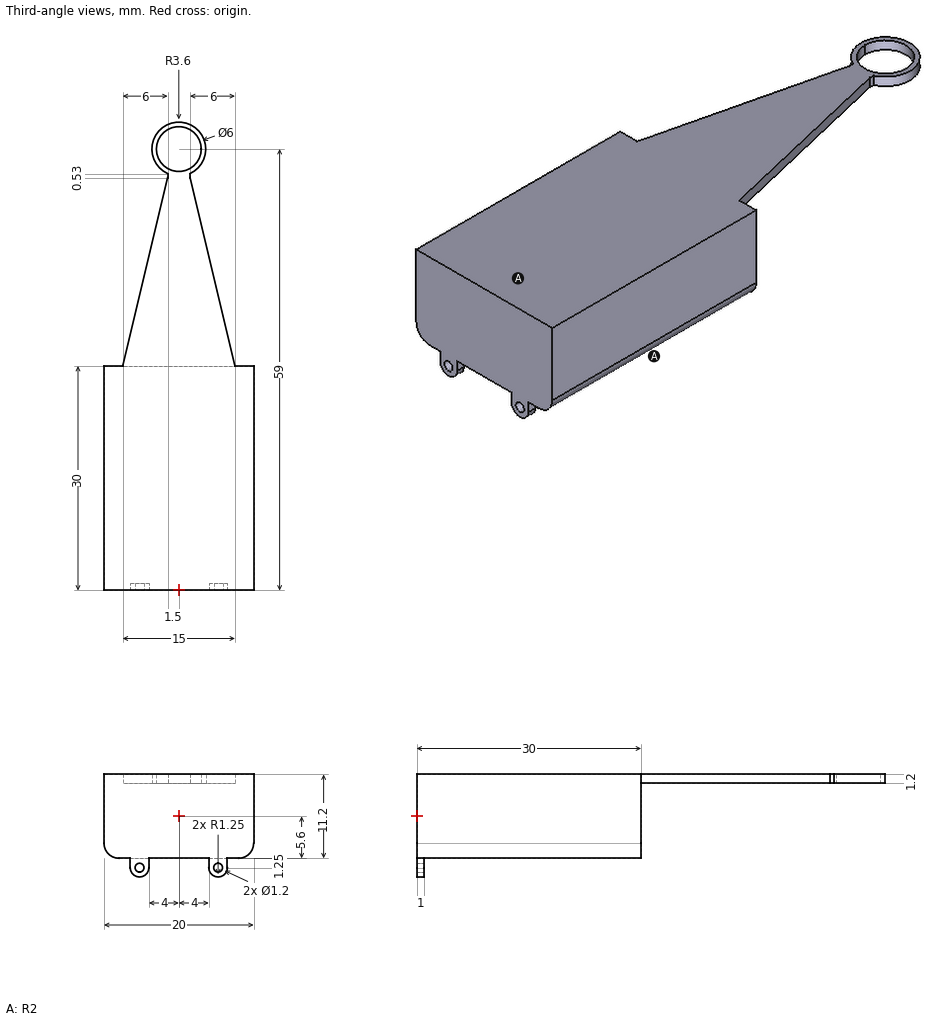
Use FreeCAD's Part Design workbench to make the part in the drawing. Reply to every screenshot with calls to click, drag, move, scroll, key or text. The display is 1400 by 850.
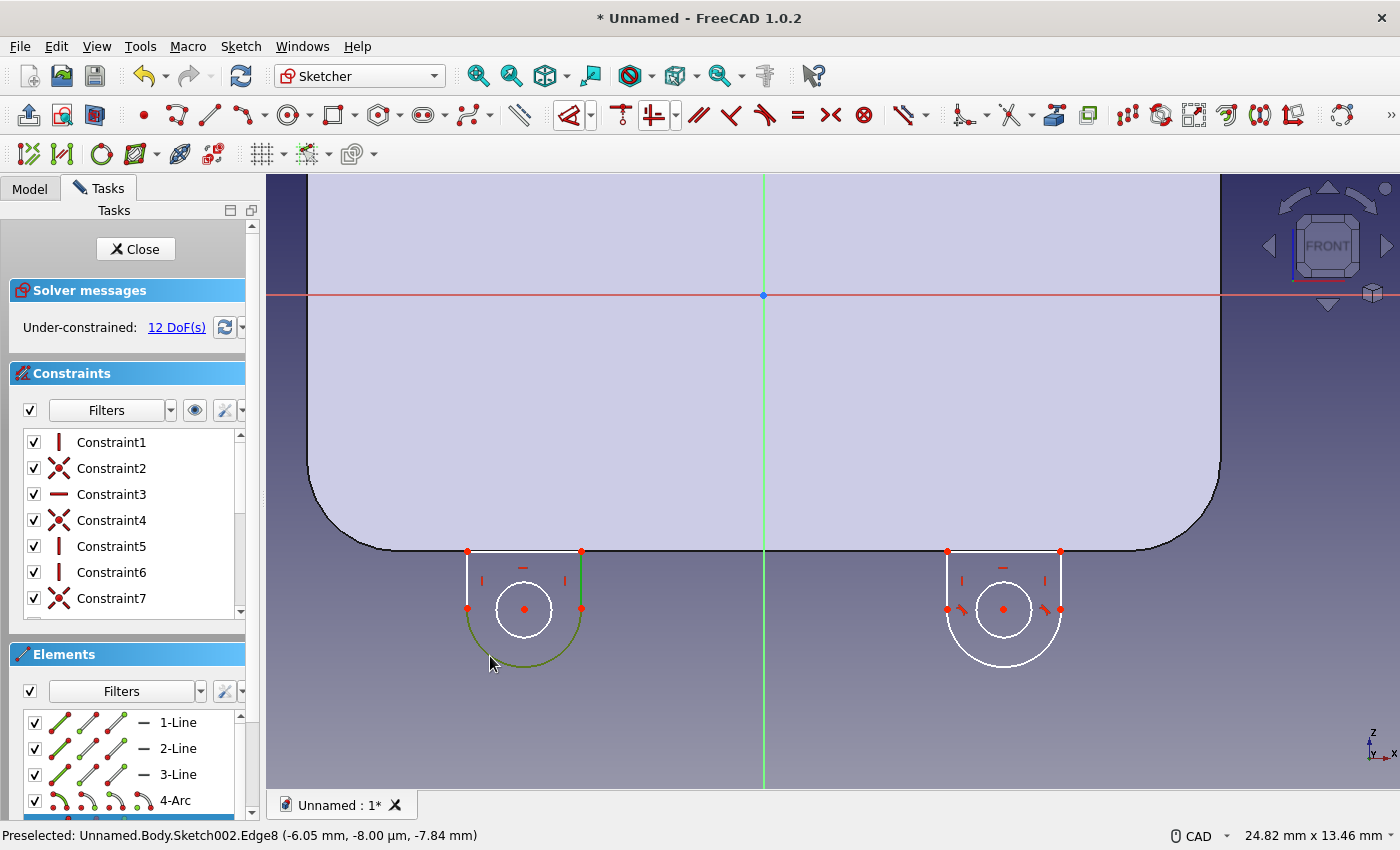
key(t)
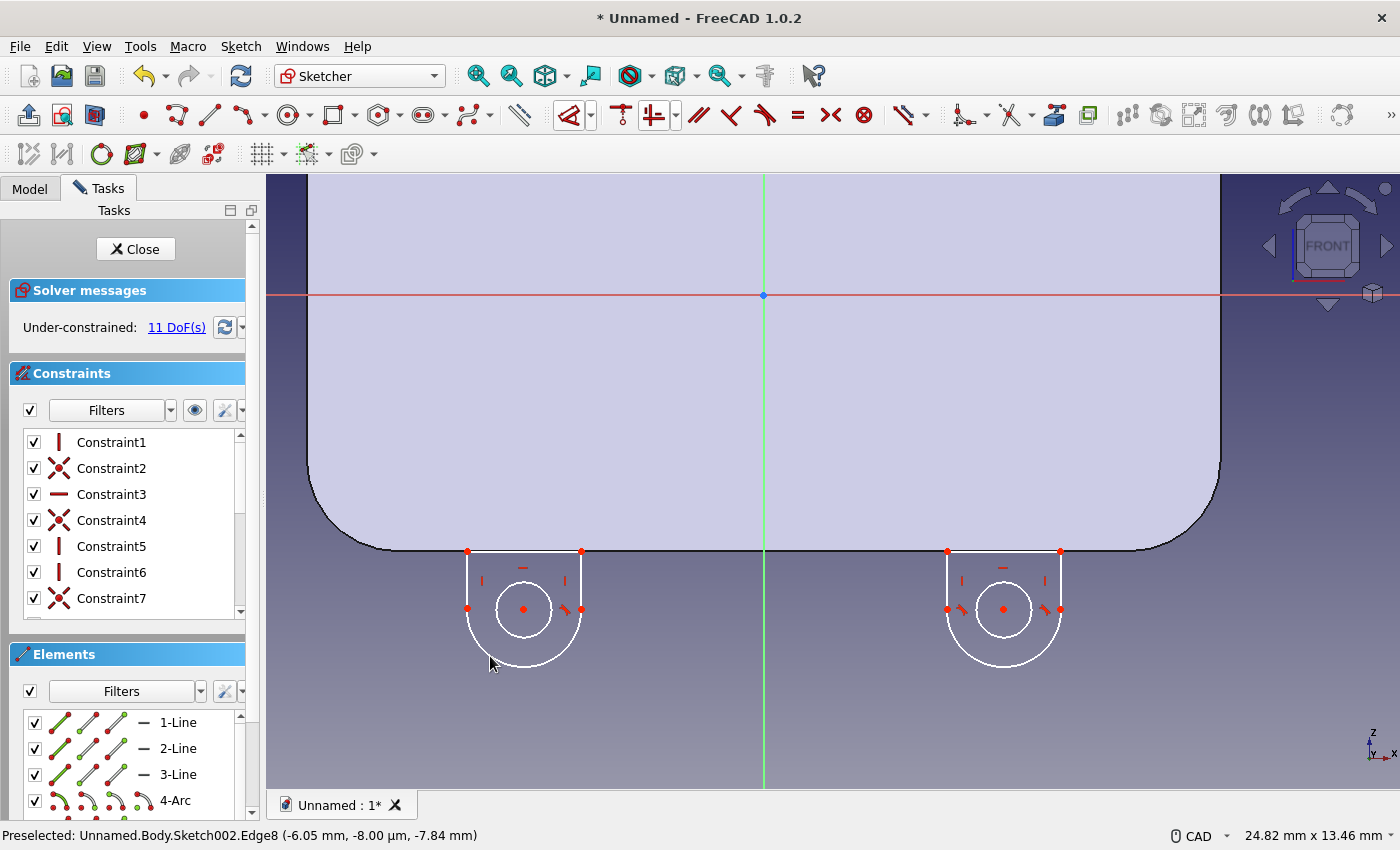
click(467, 569)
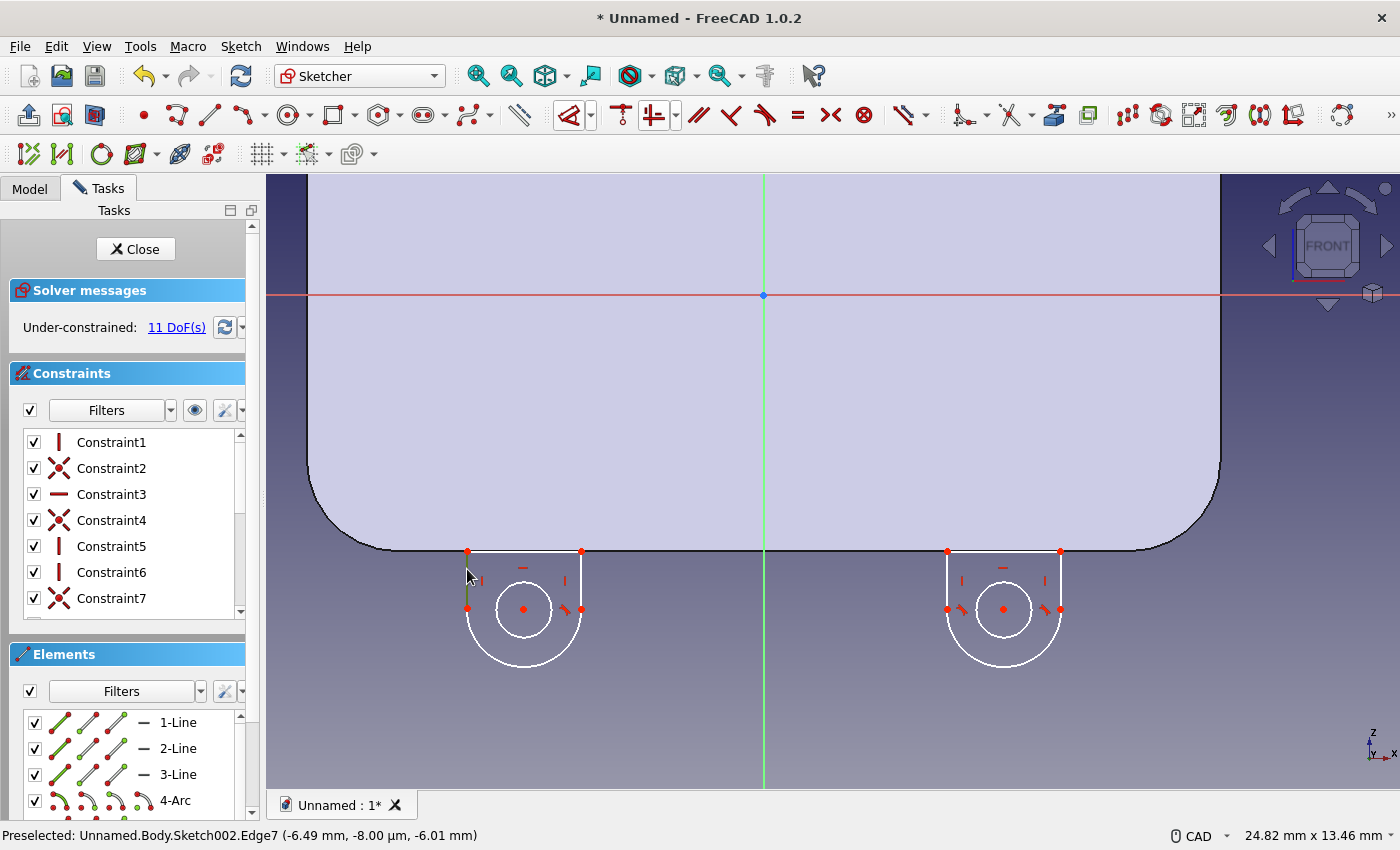
click(490, 656)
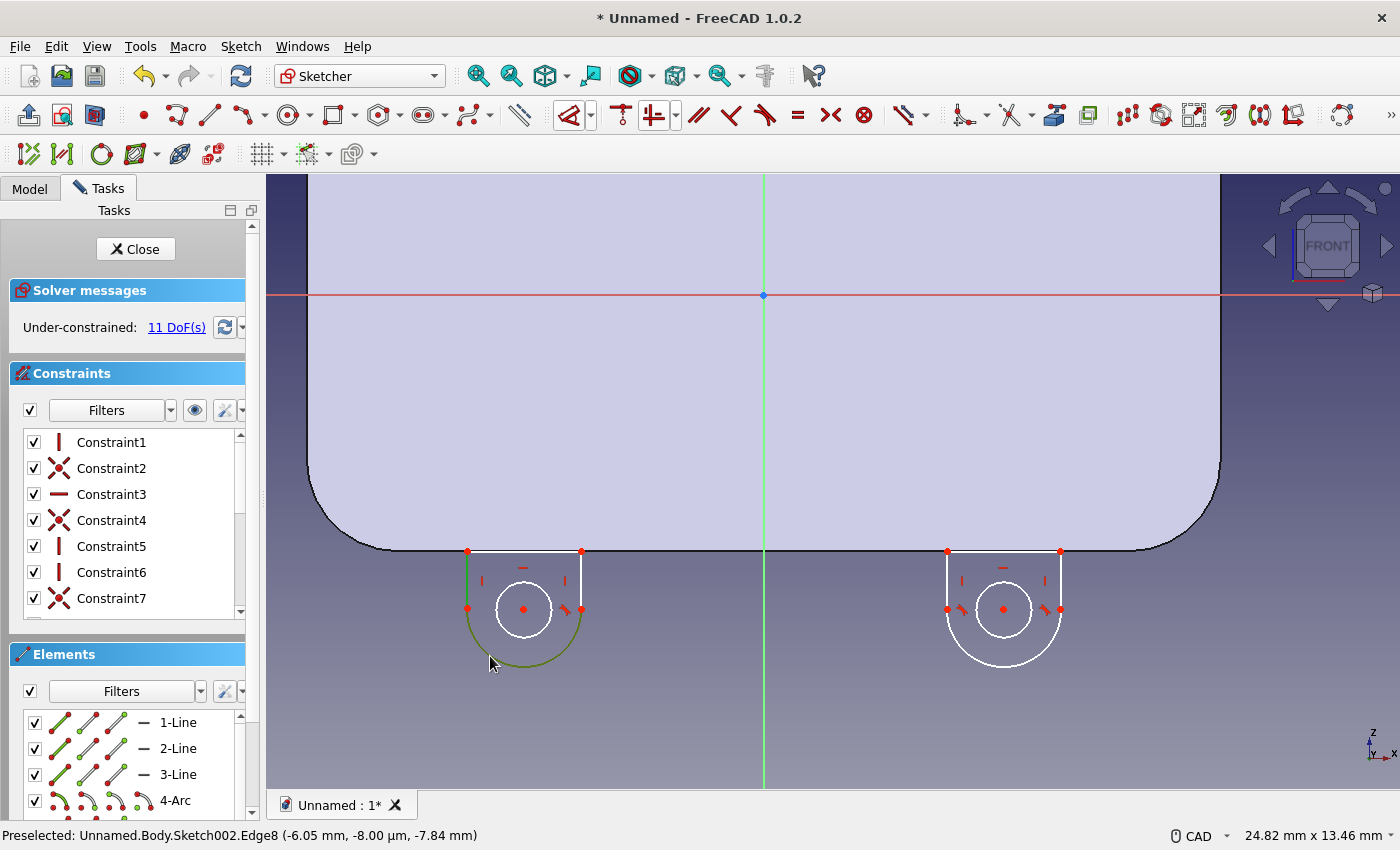
key(t)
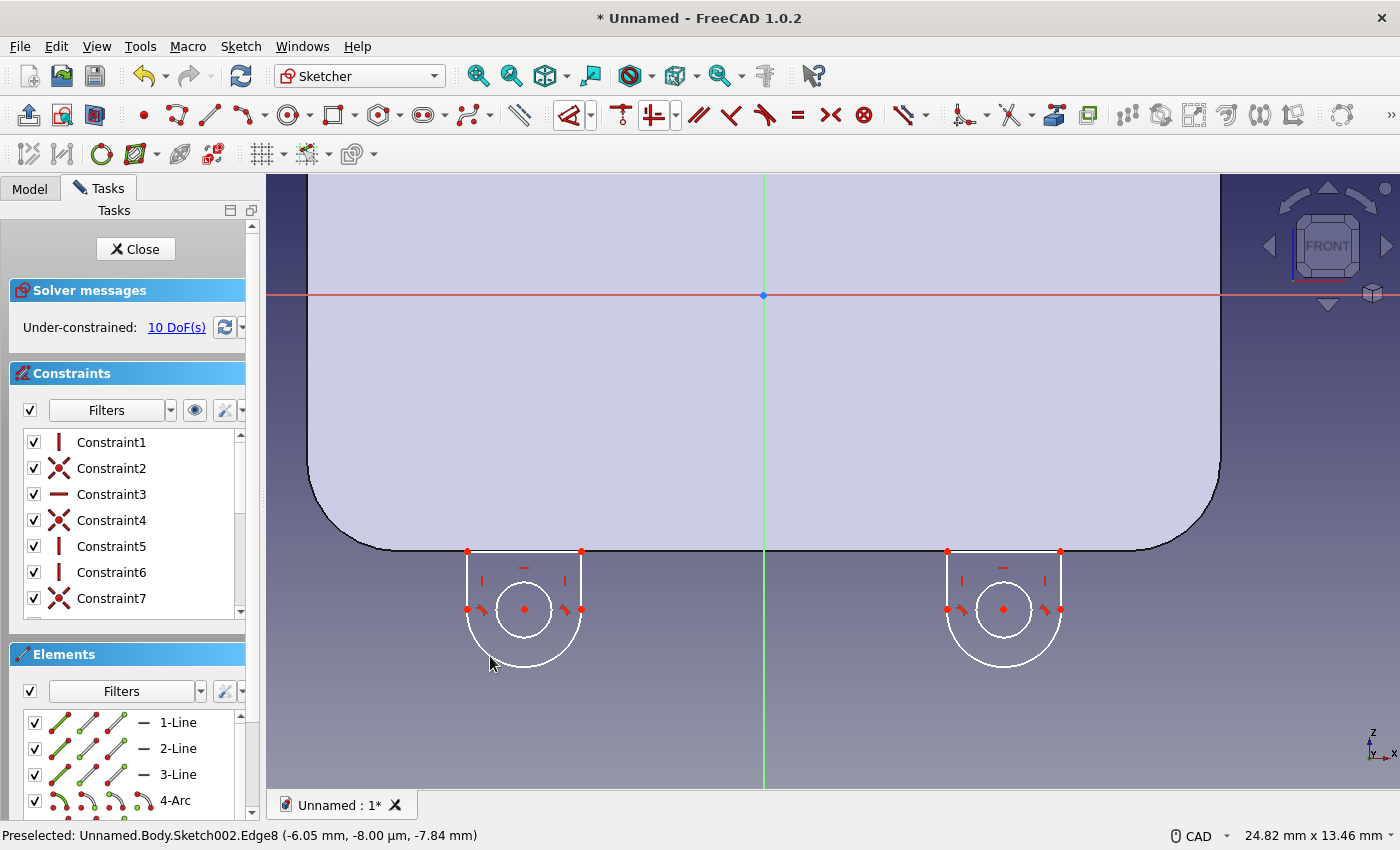
click(970, 656)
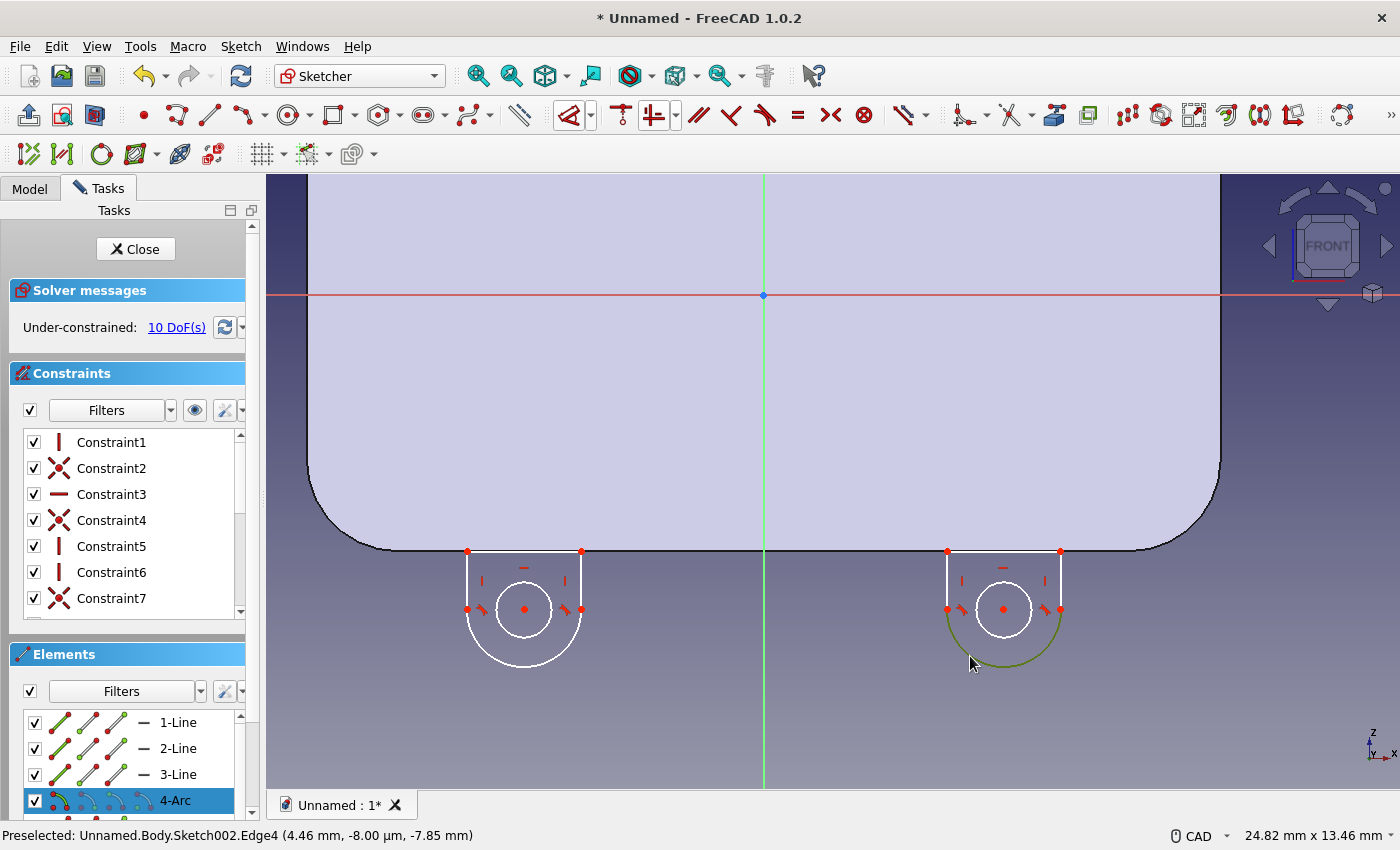
click(491, 656)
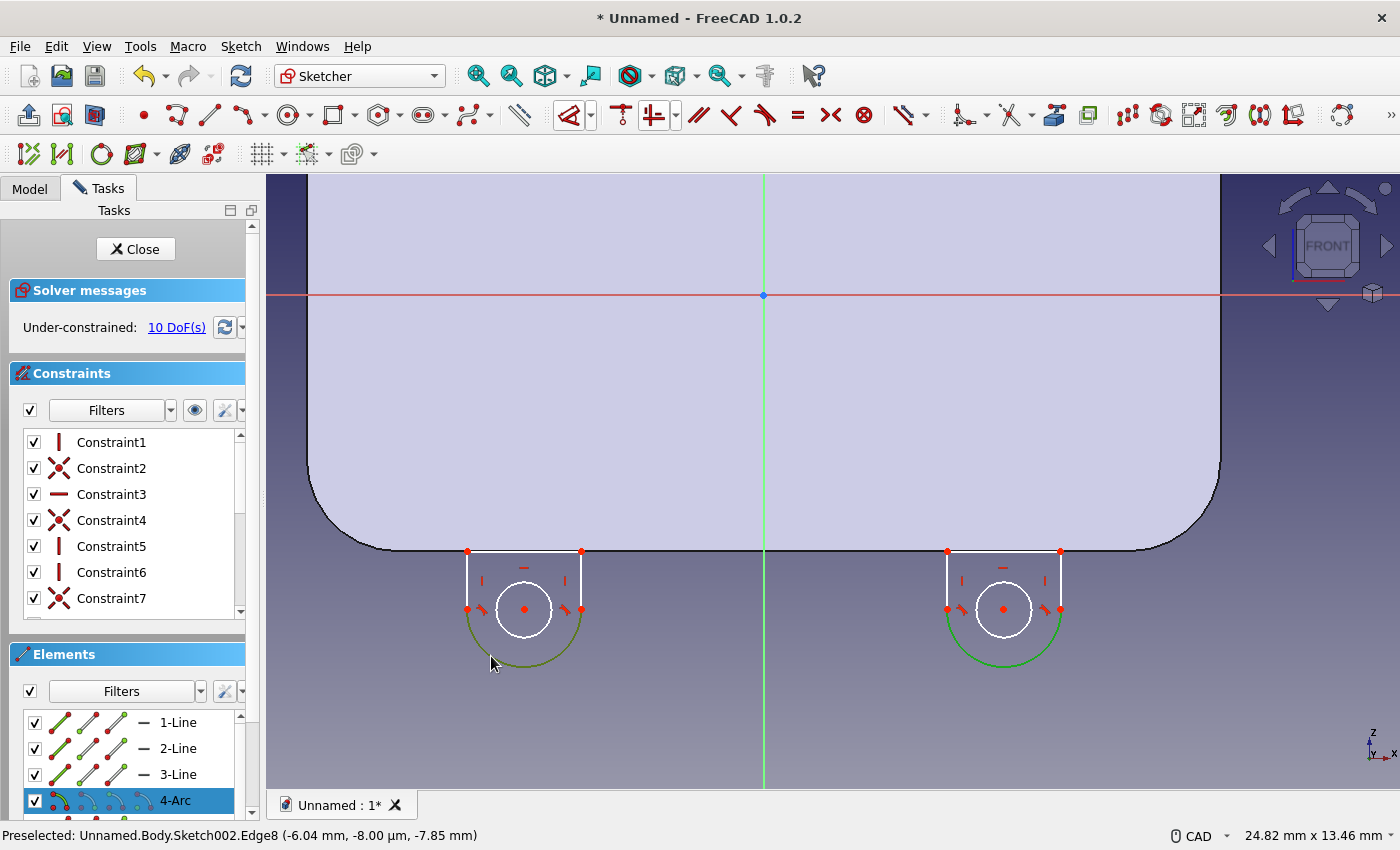
key(e)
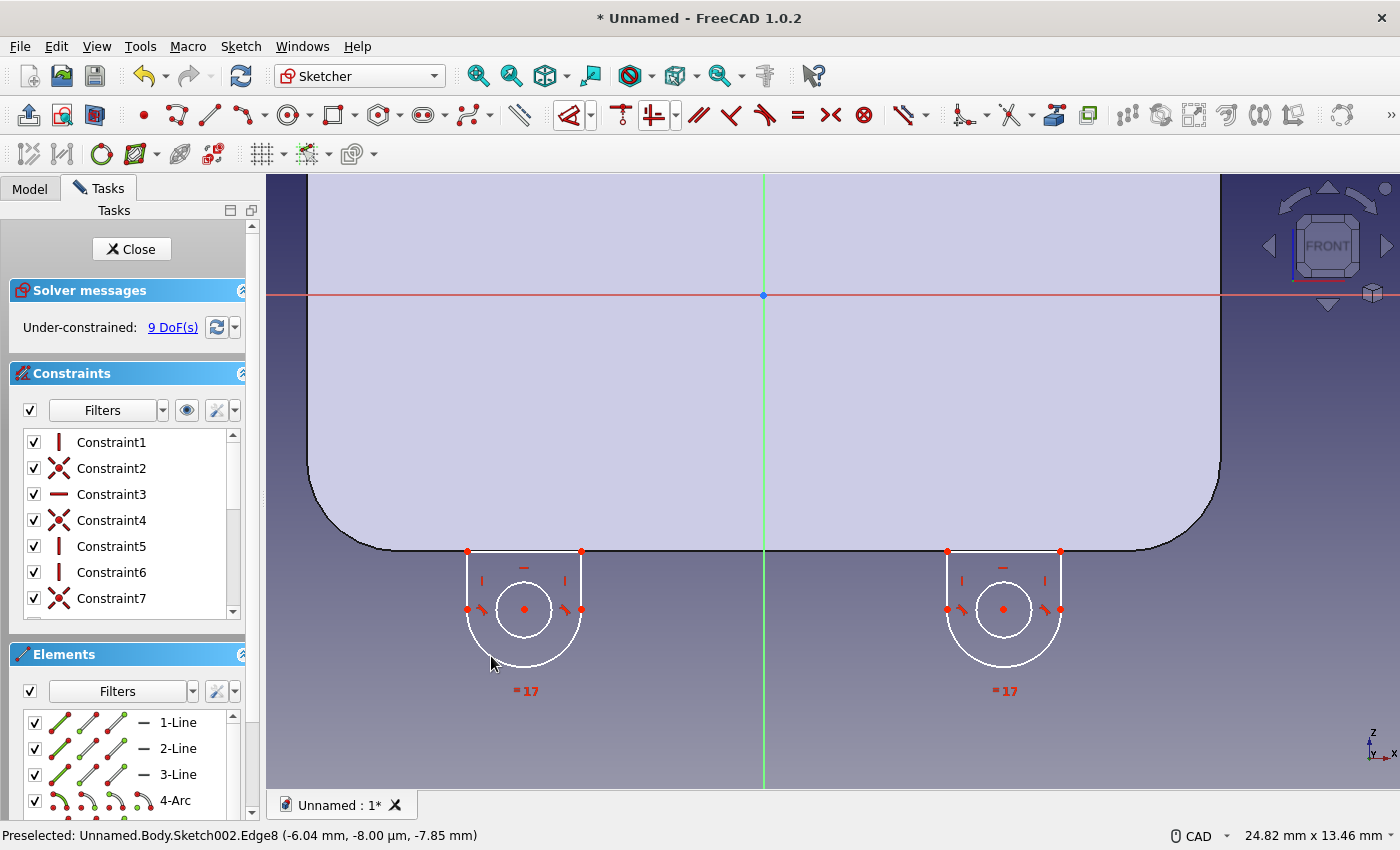
click(1023, 590)